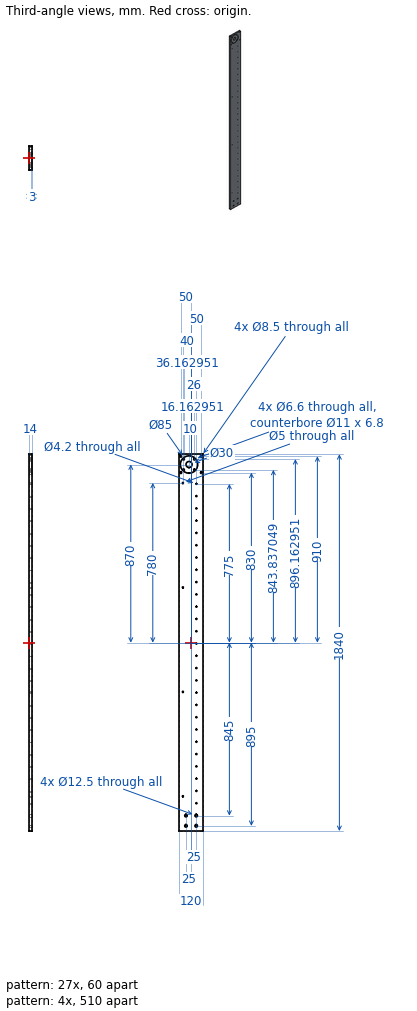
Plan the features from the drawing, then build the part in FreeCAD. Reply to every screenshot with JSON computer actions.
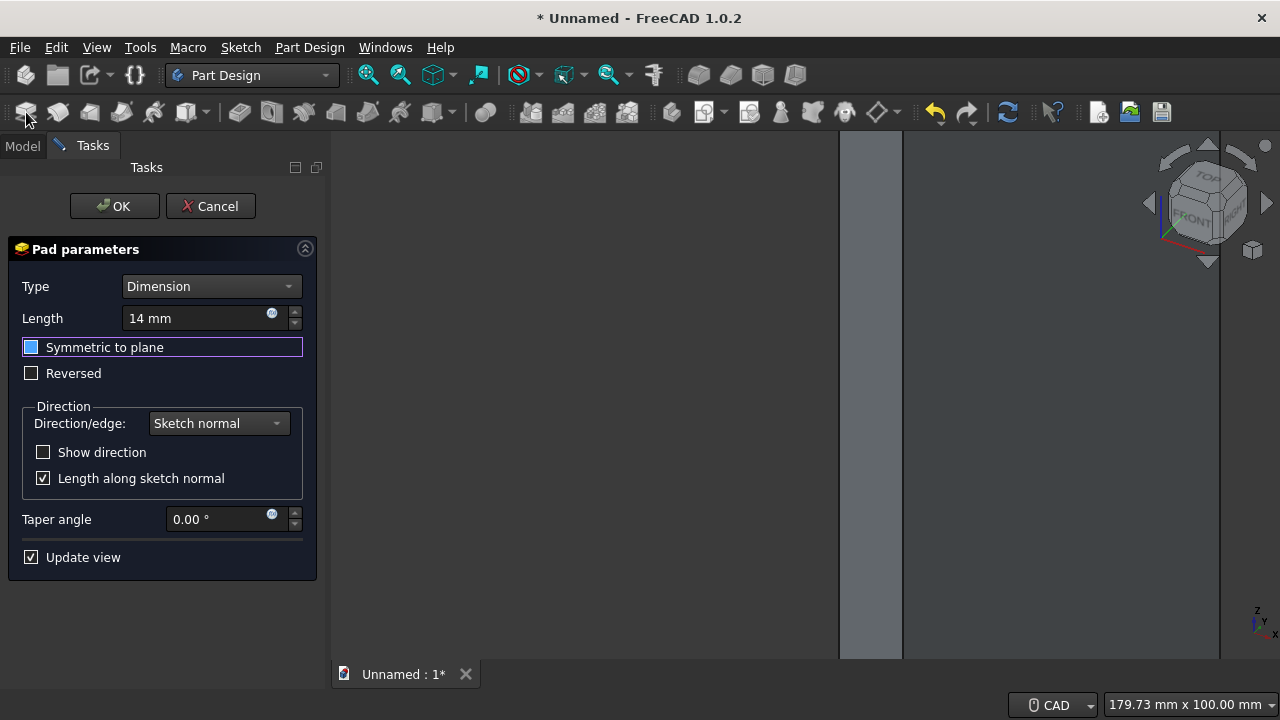
{"action": "left_click", "coordinate": [115, 206]}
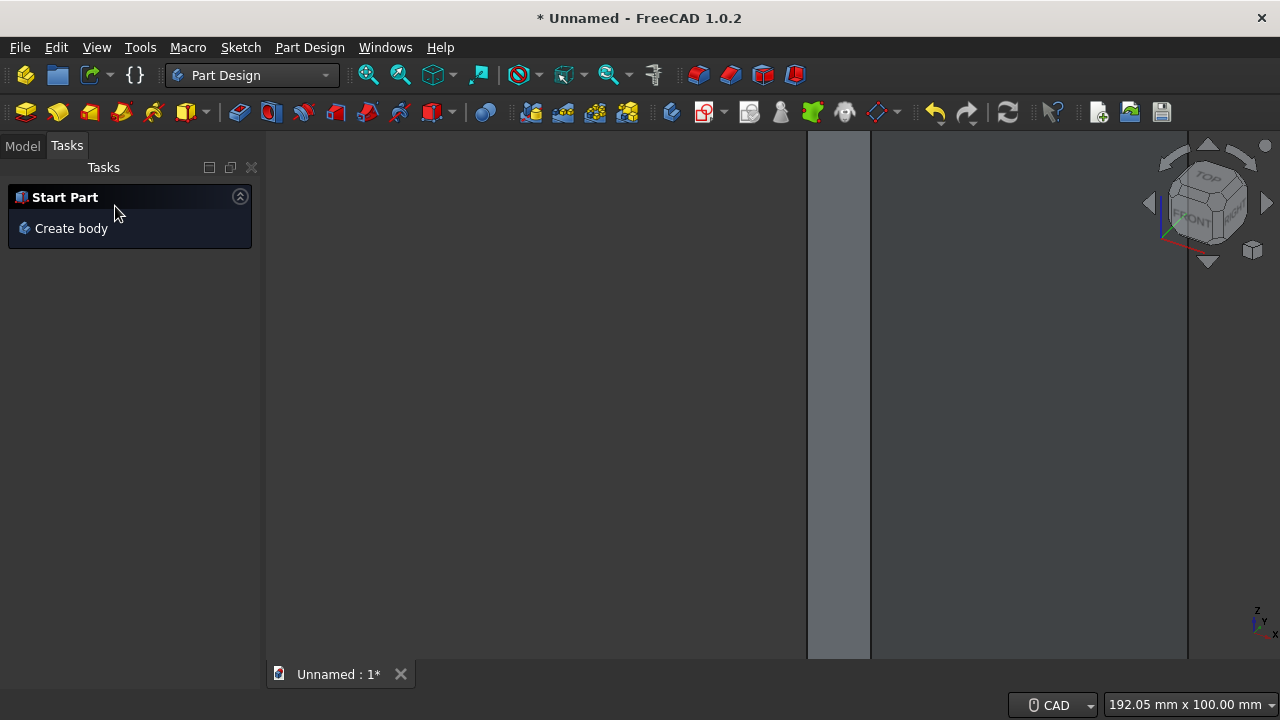
{"action": "left_click", "coordinate": [370, 76]}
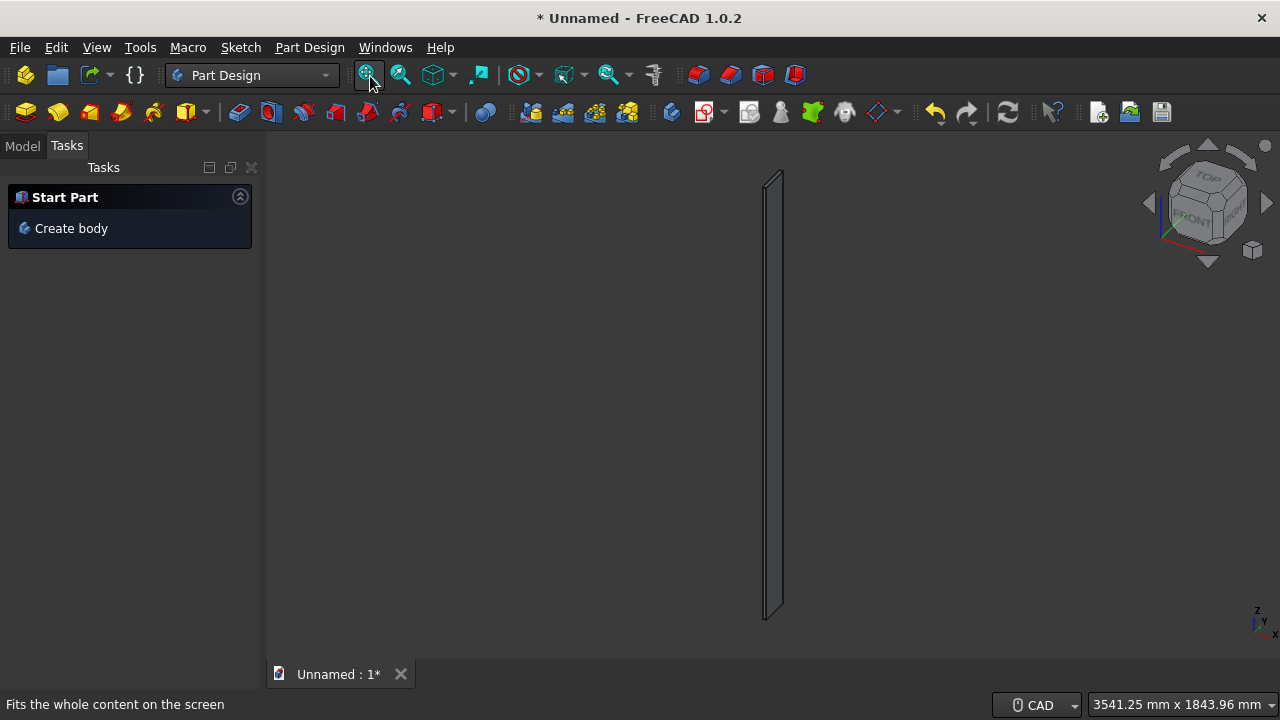
{"action": "left_click", "coordinate": [704, 112]}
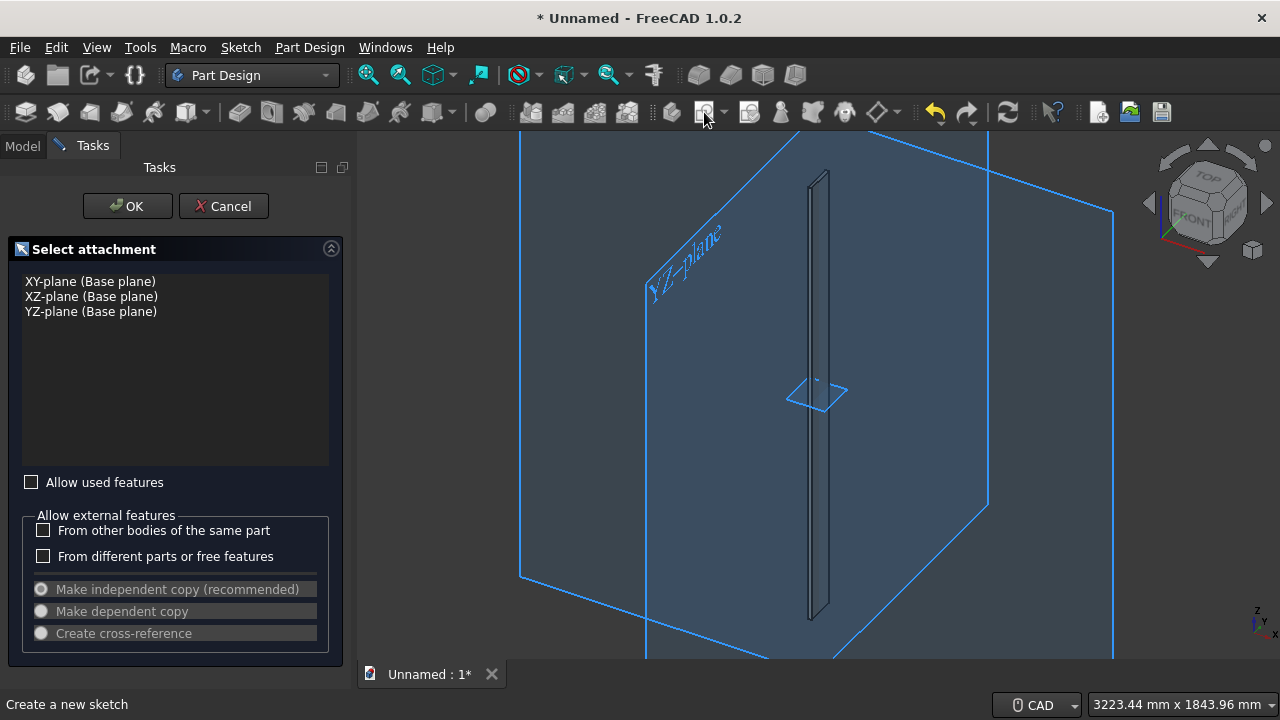
{"action": "left_click", "coordinate": [82, 312]}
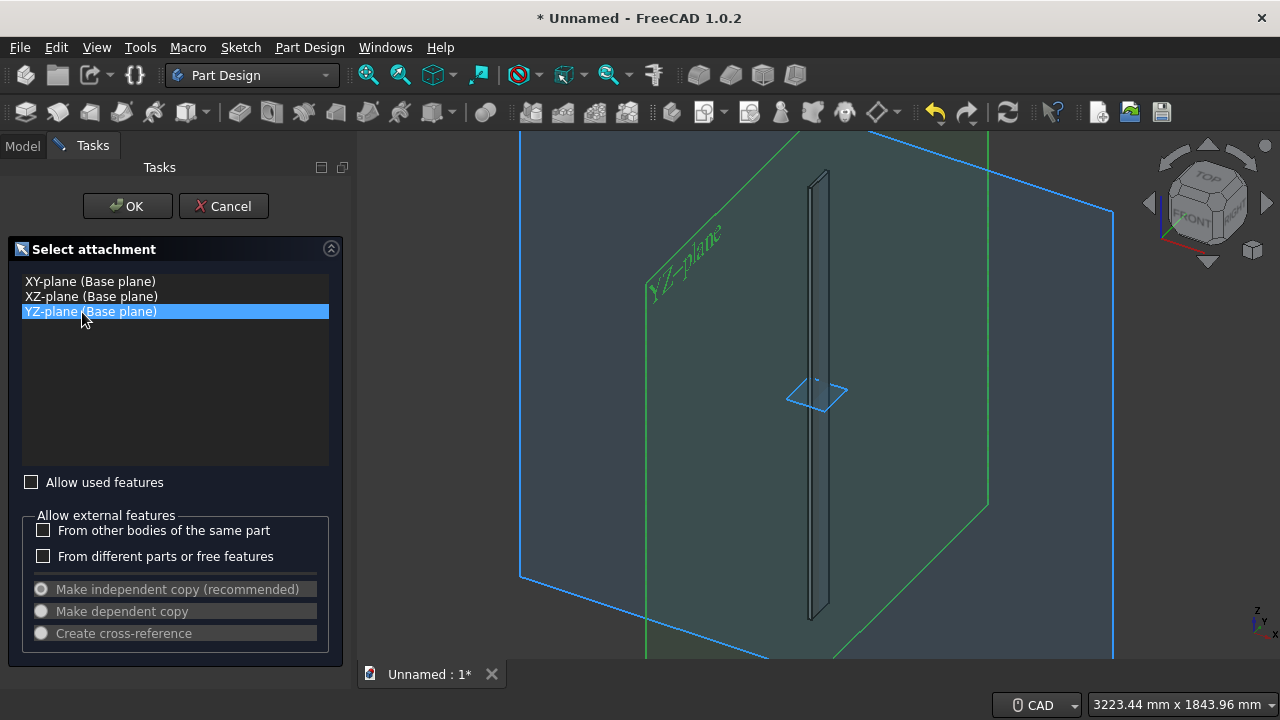
{"action": "left_click", "coordinate": [128, 206]}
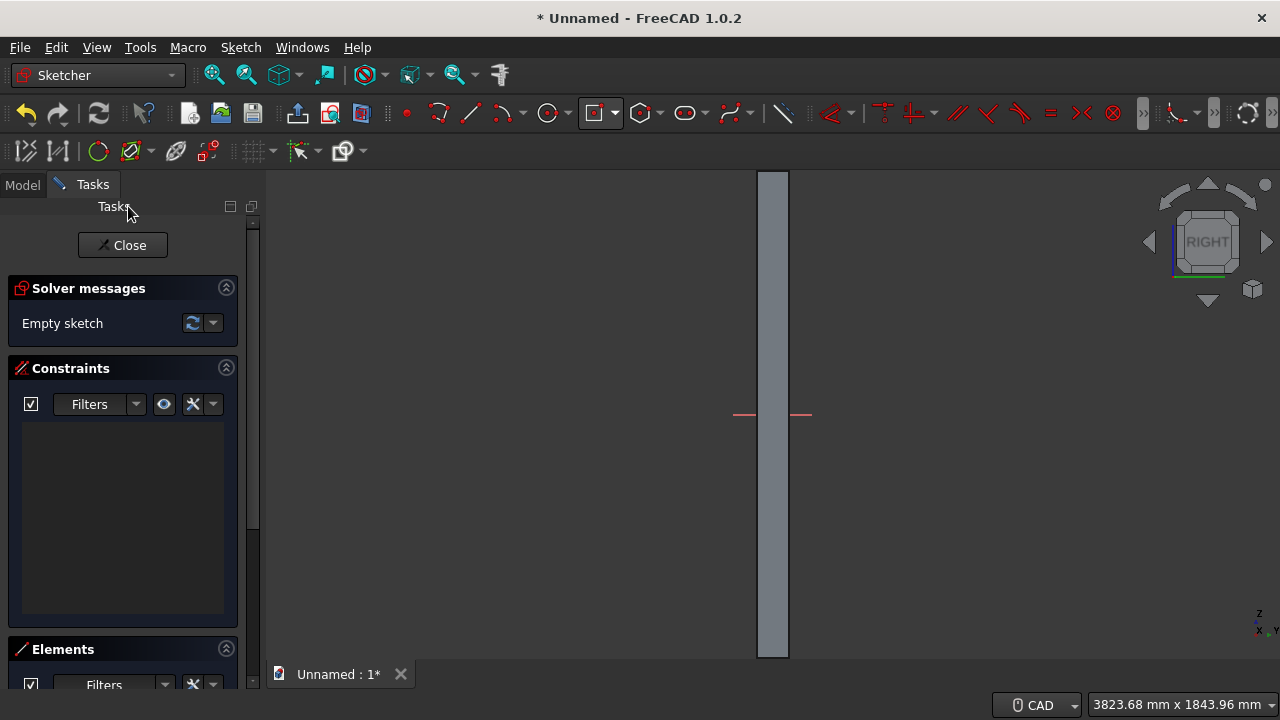
{"action": "left_click", "coordinate": [362, 114]}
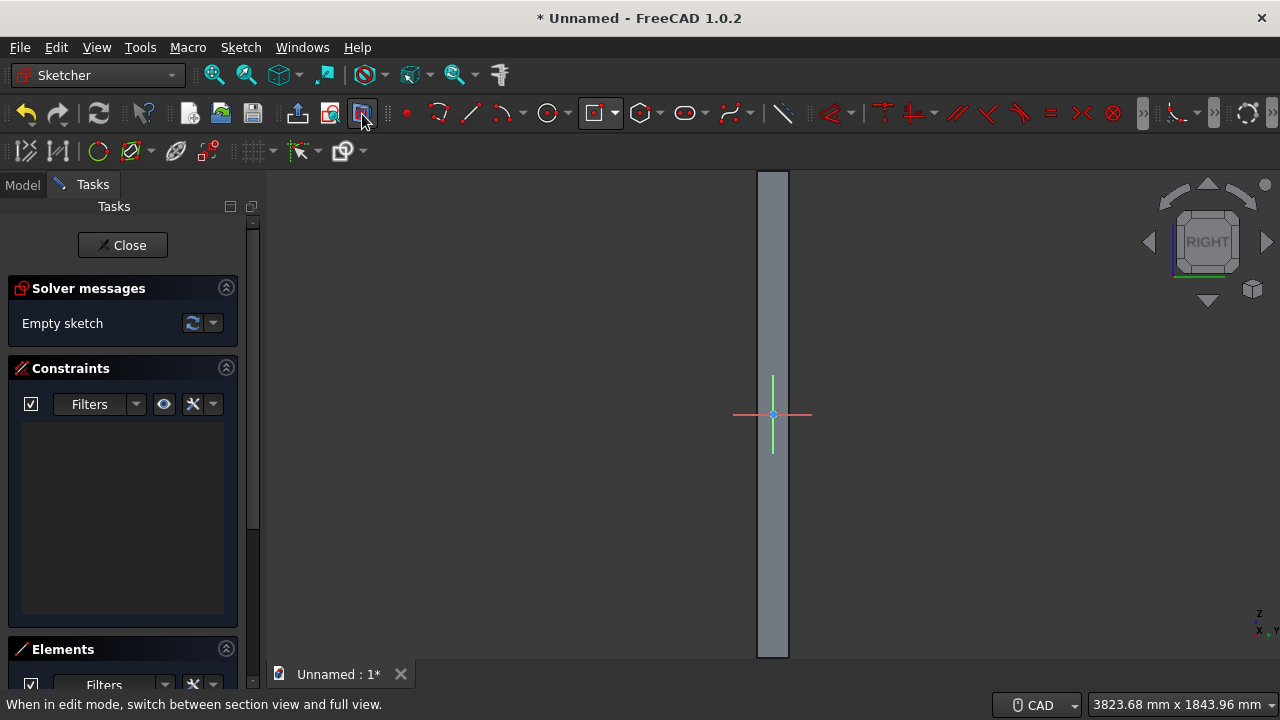
{"action": "scroll", "coordinate": [704, 414], "scroll_direction": "down", "scroll_amount": 5}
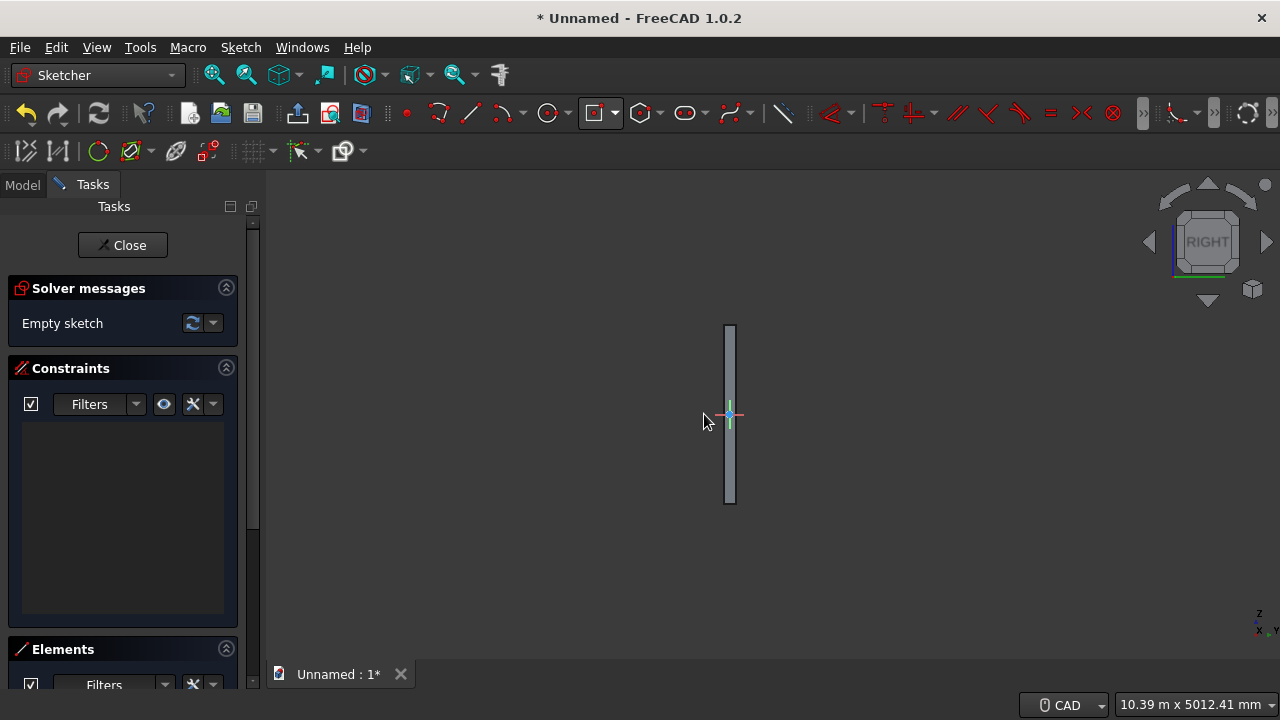
{"action": "scroll", "coordinate": [730, 325], "scroll_direction": "up", "scroll_amount": 15}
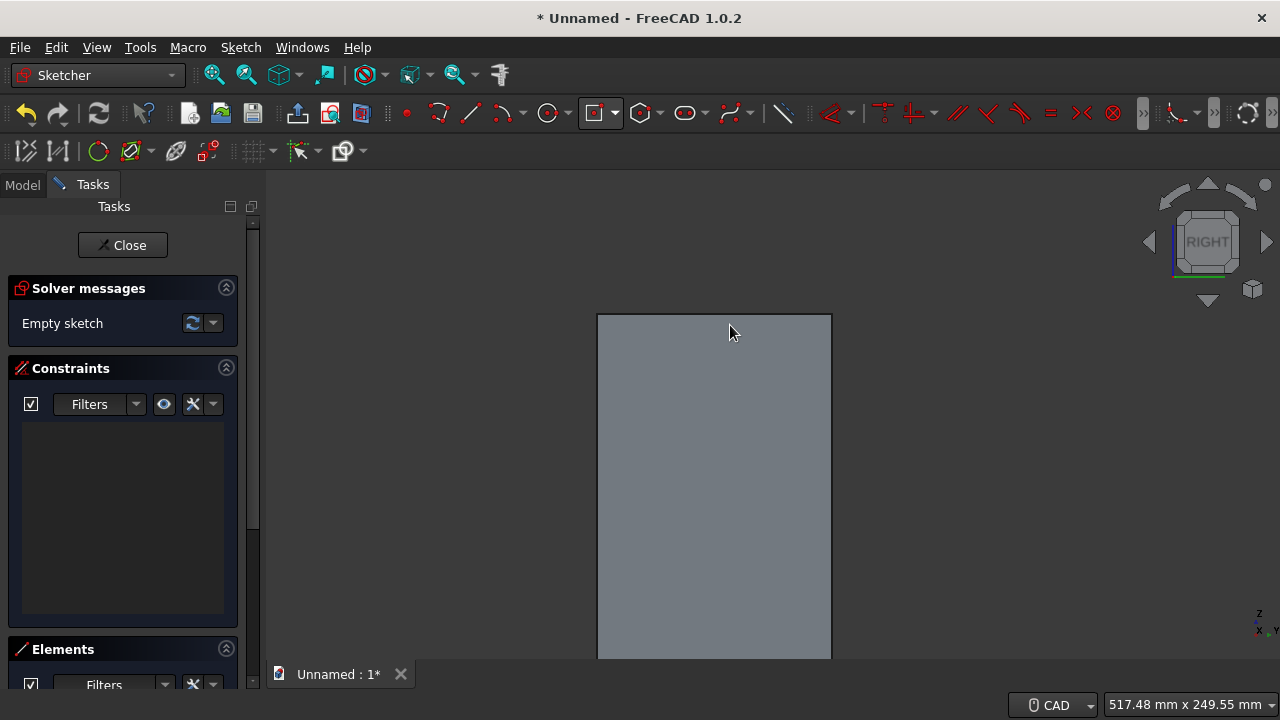
{"action": "scroll", "coordinate": [689, 410], "scroll_direction": "up", "scroll_amount": 5}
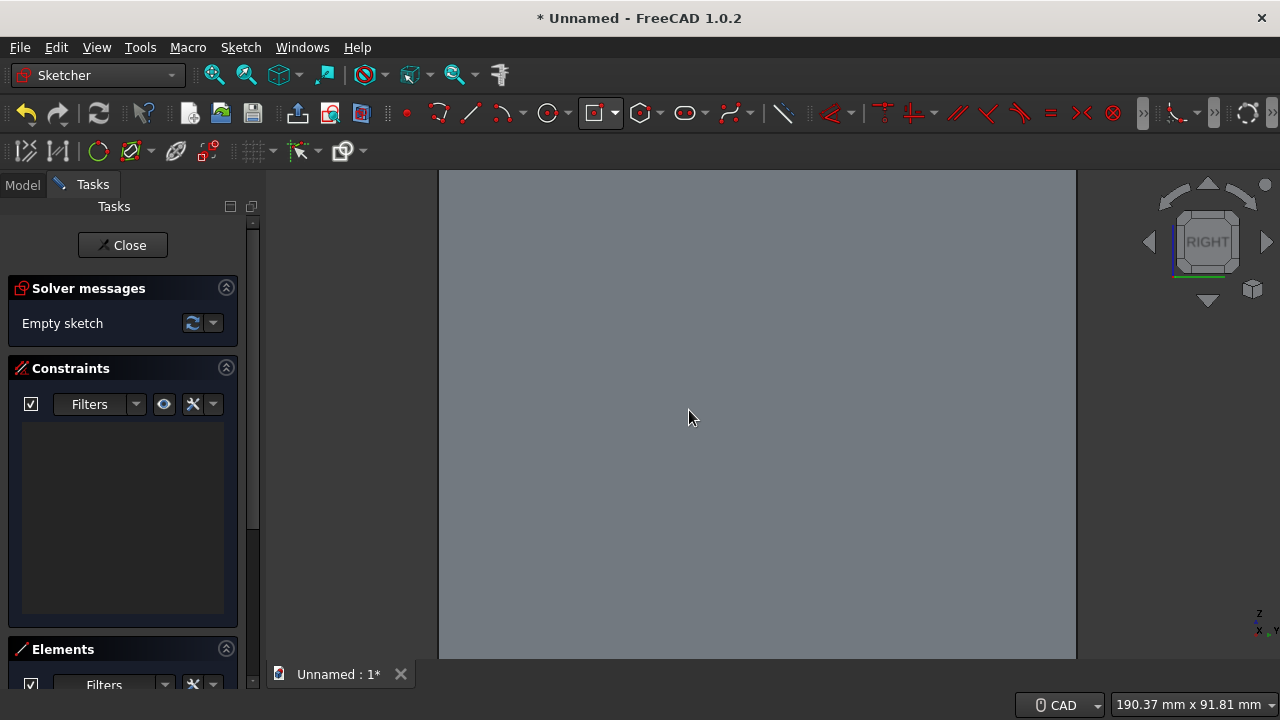
{"action": "left_click", "coordinate": [548, 114]}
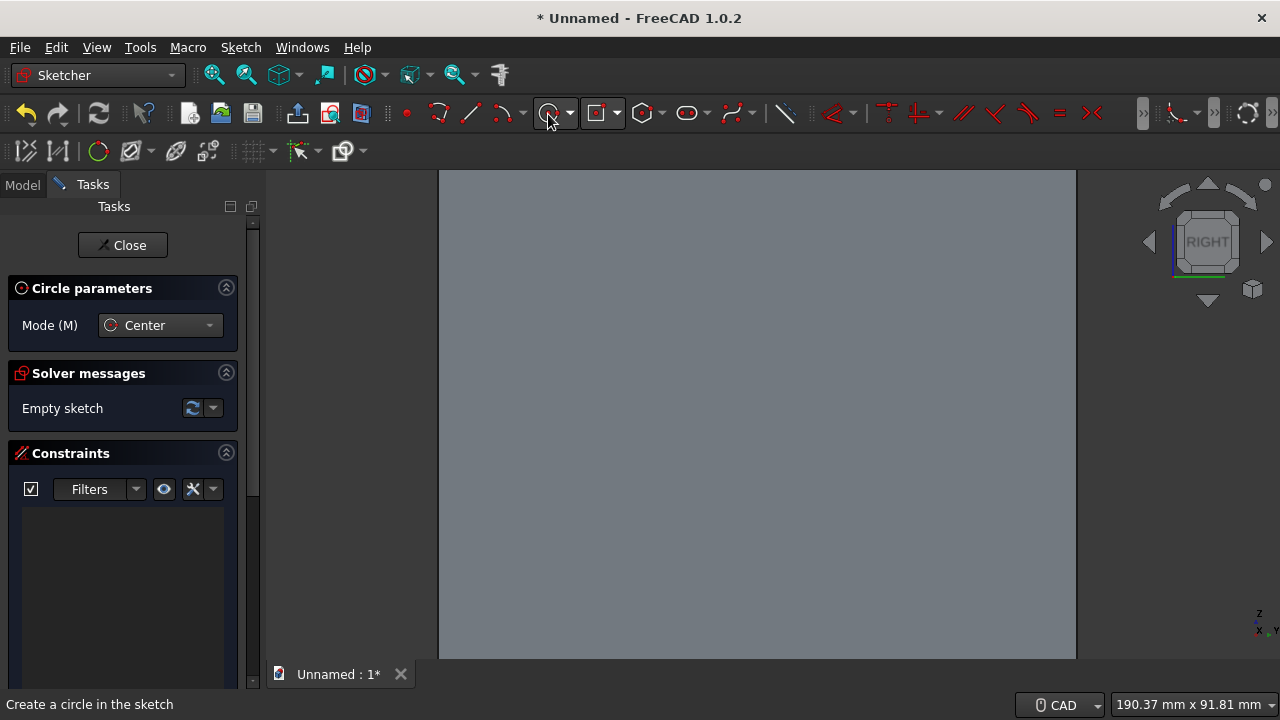
{"action": "scroll", "coordinate": [843, 275], "scroll_direction": "up", "scroll_amount": 2}